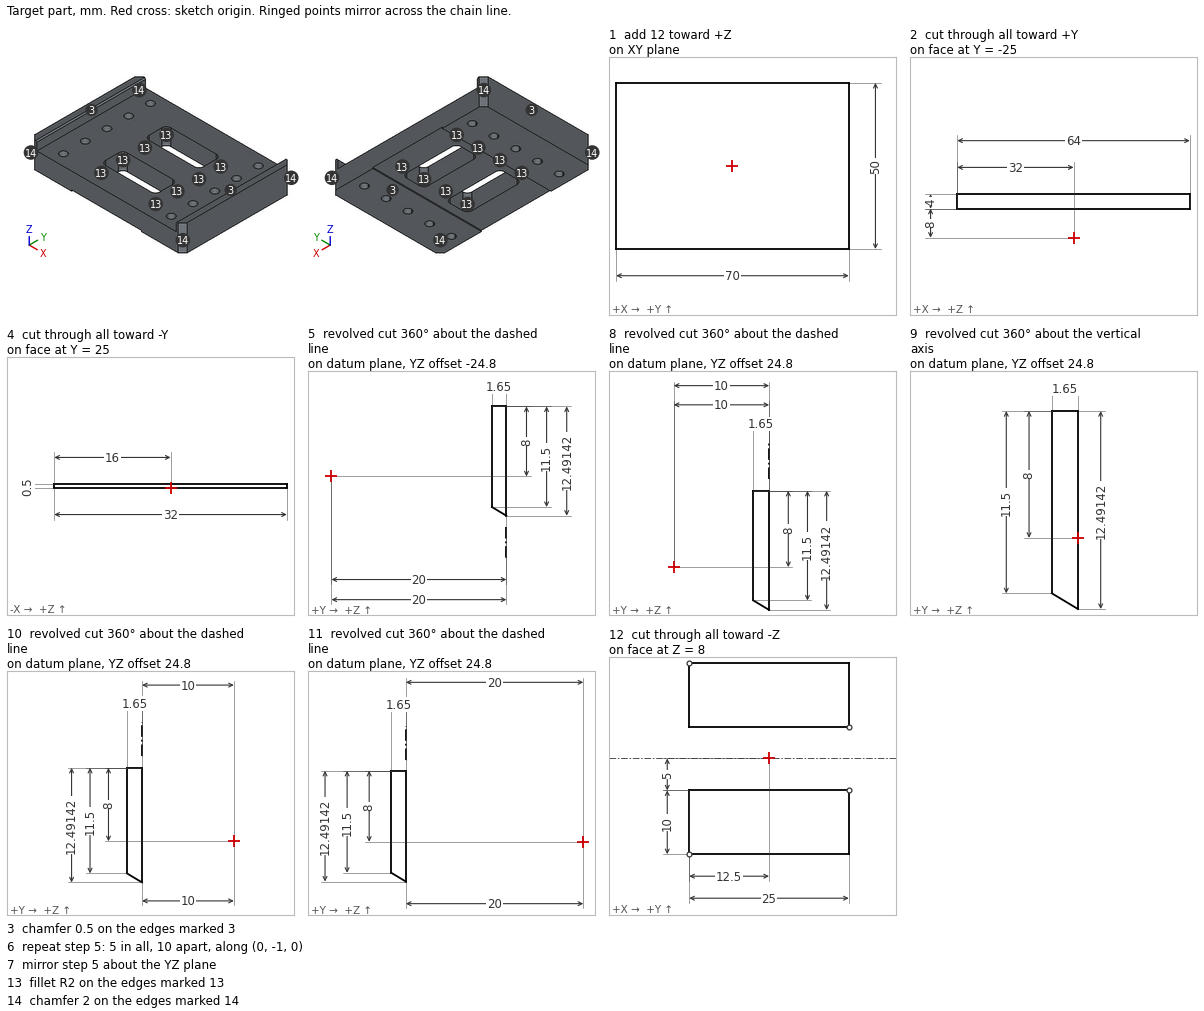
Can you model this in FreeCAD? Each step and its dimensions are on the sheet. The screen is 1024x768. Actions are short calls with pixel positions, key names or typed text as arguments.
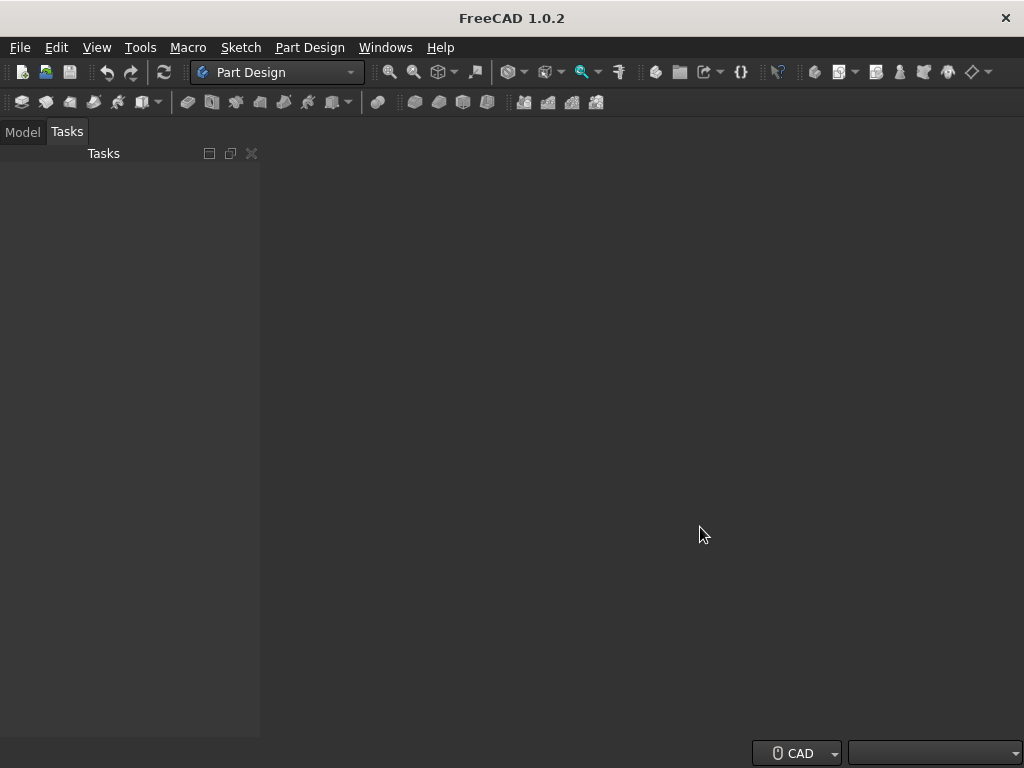
key(ctrl+n)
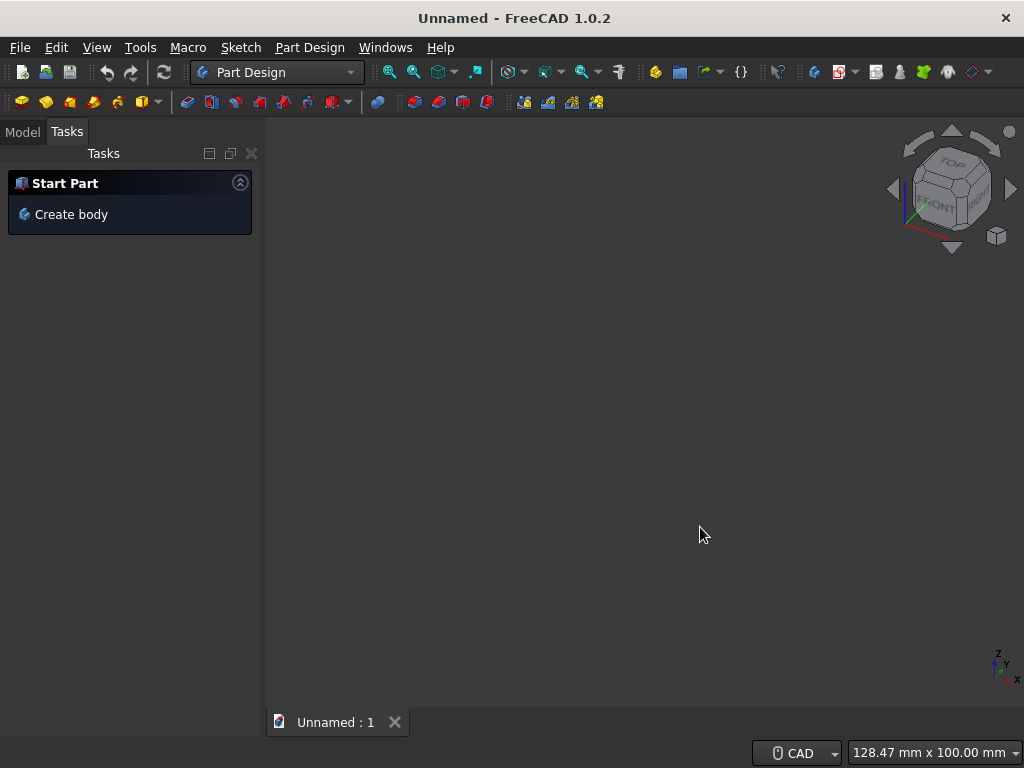
click(840, 72)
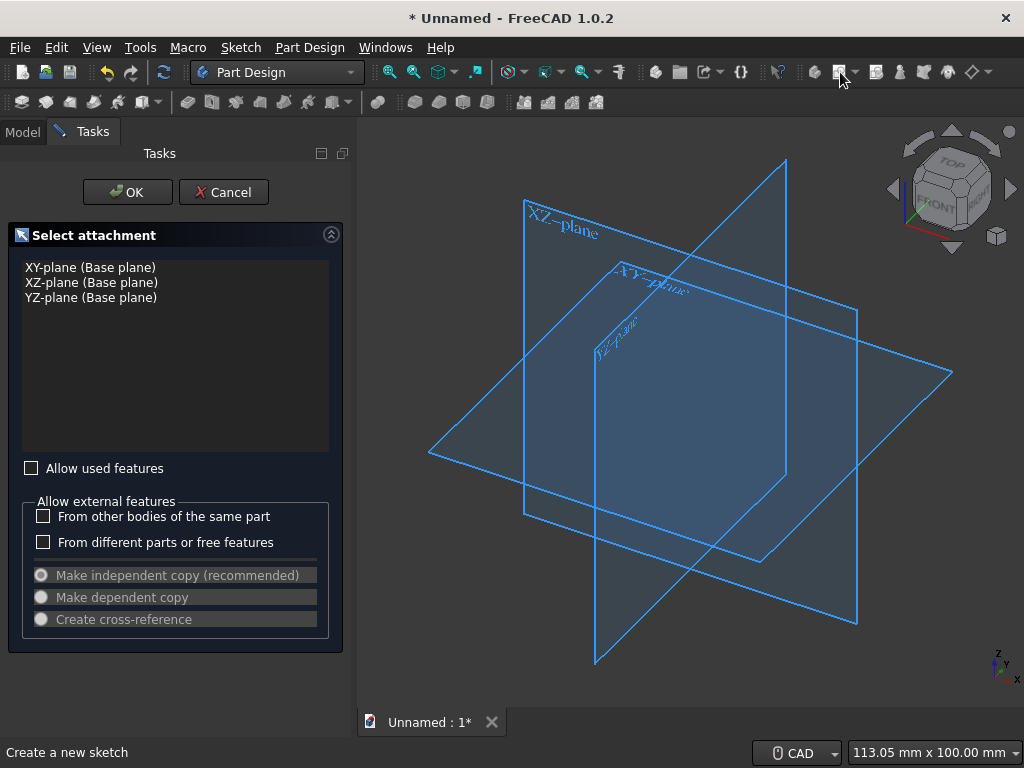
click(82, 268)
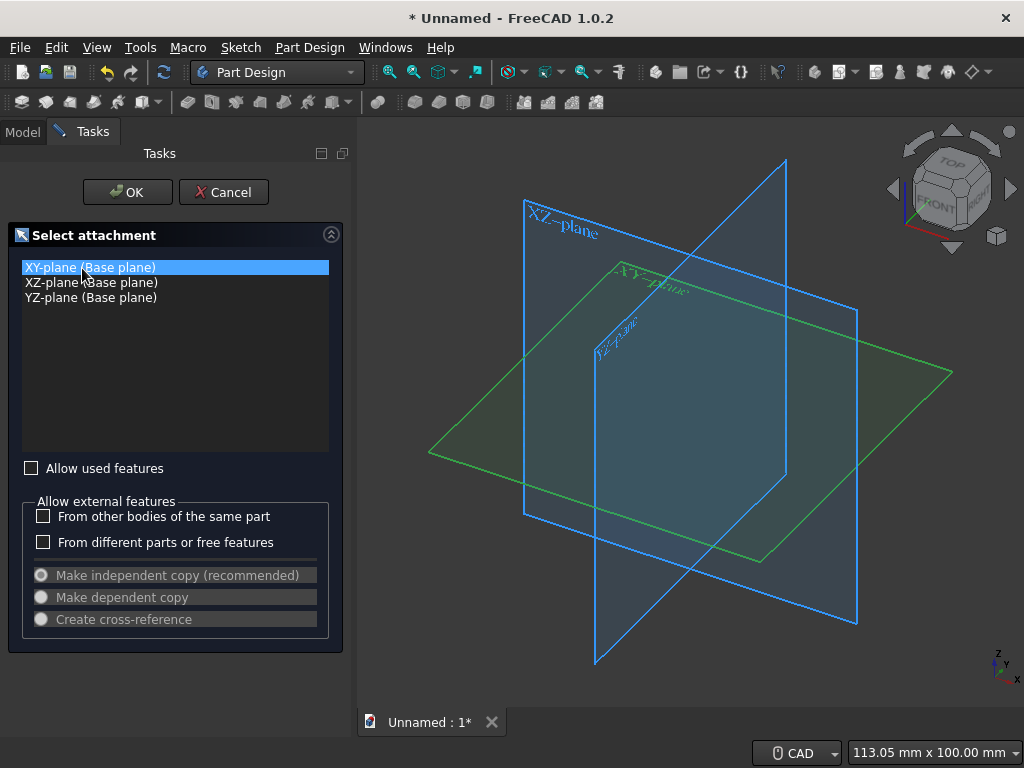
click(128, 192)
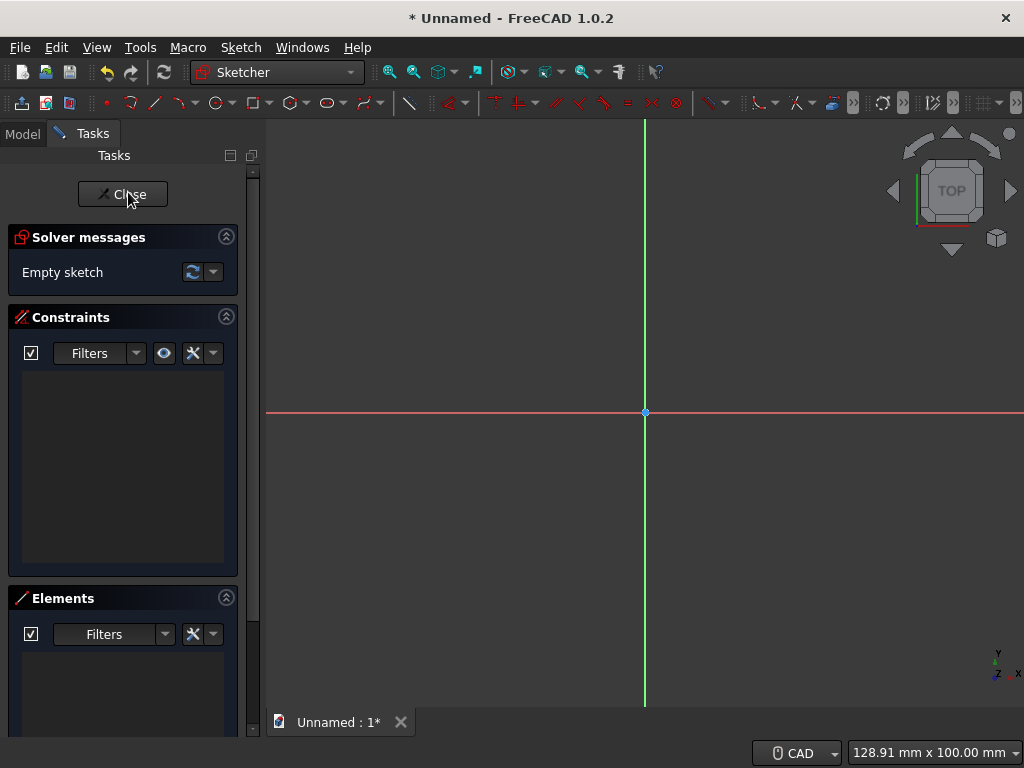
scroll(294, 413, down, 1)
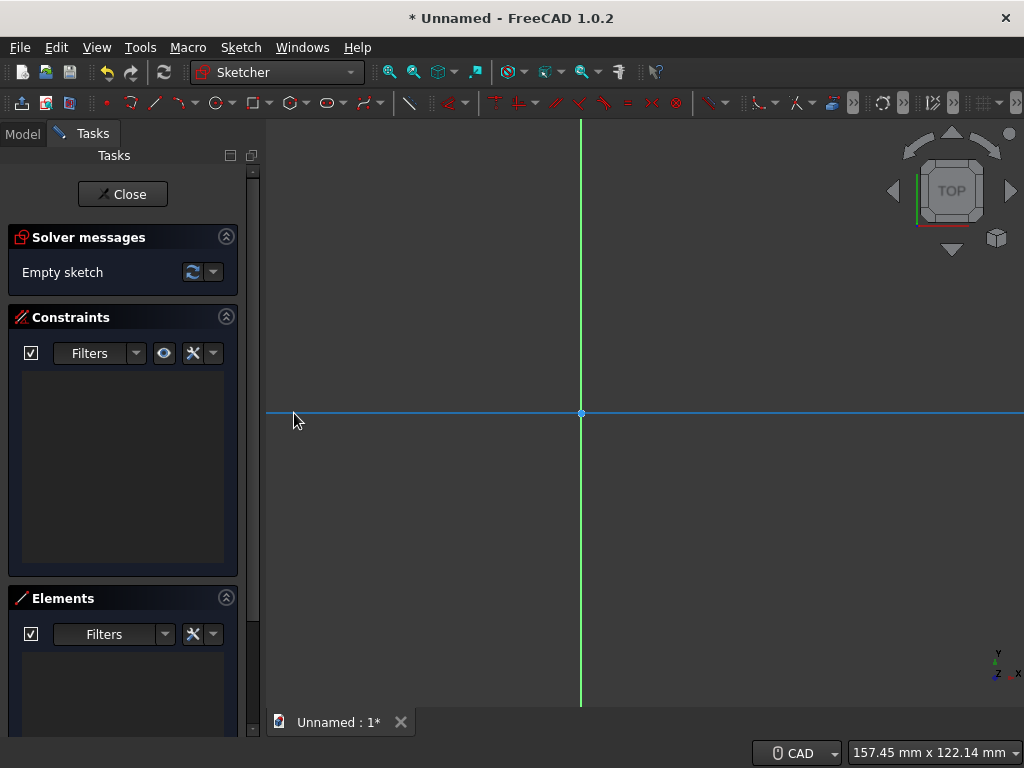
key(g)
key(v)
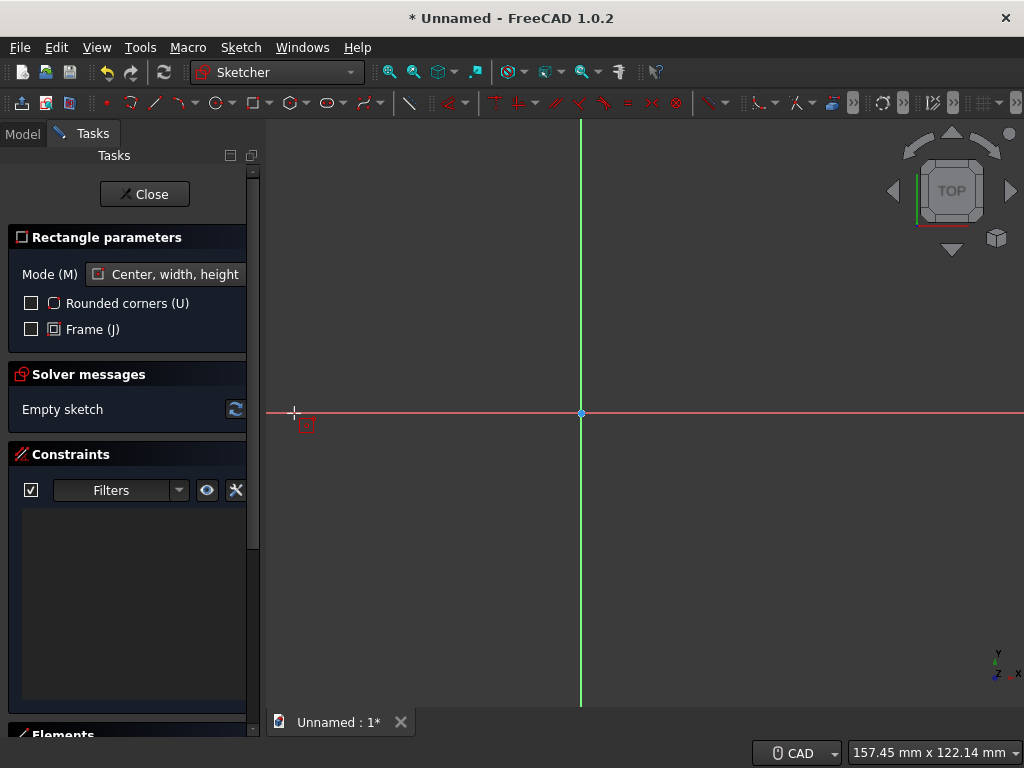
click(581, 413)
click(750, 293)
key(Escape)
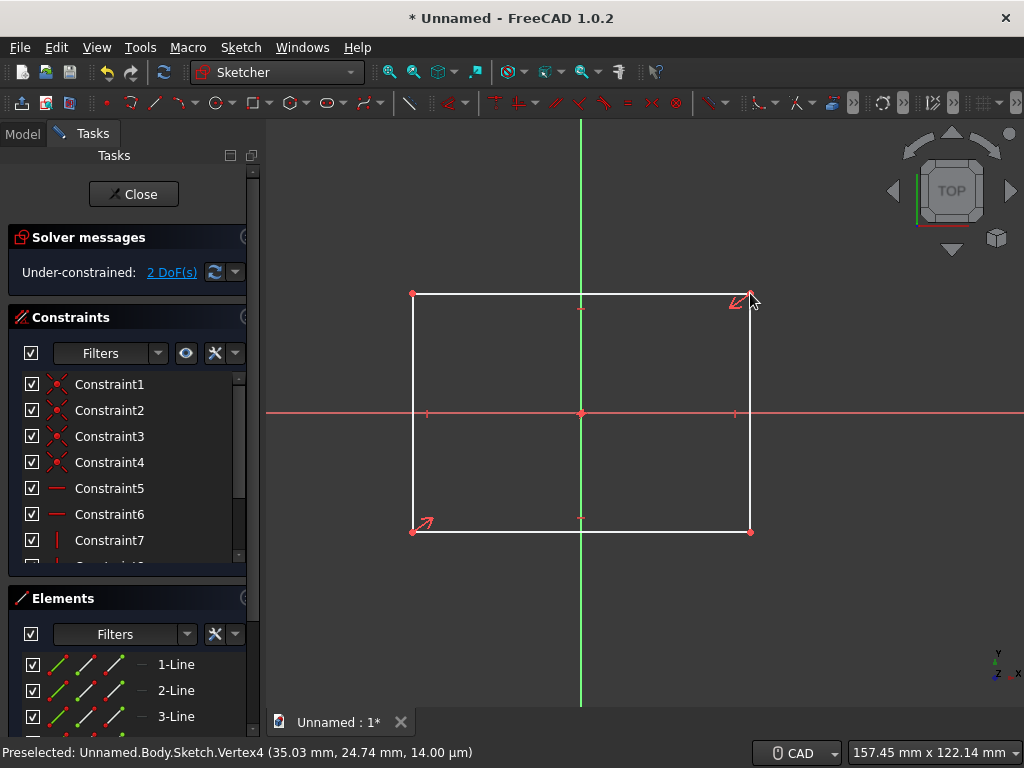
click(514, 532)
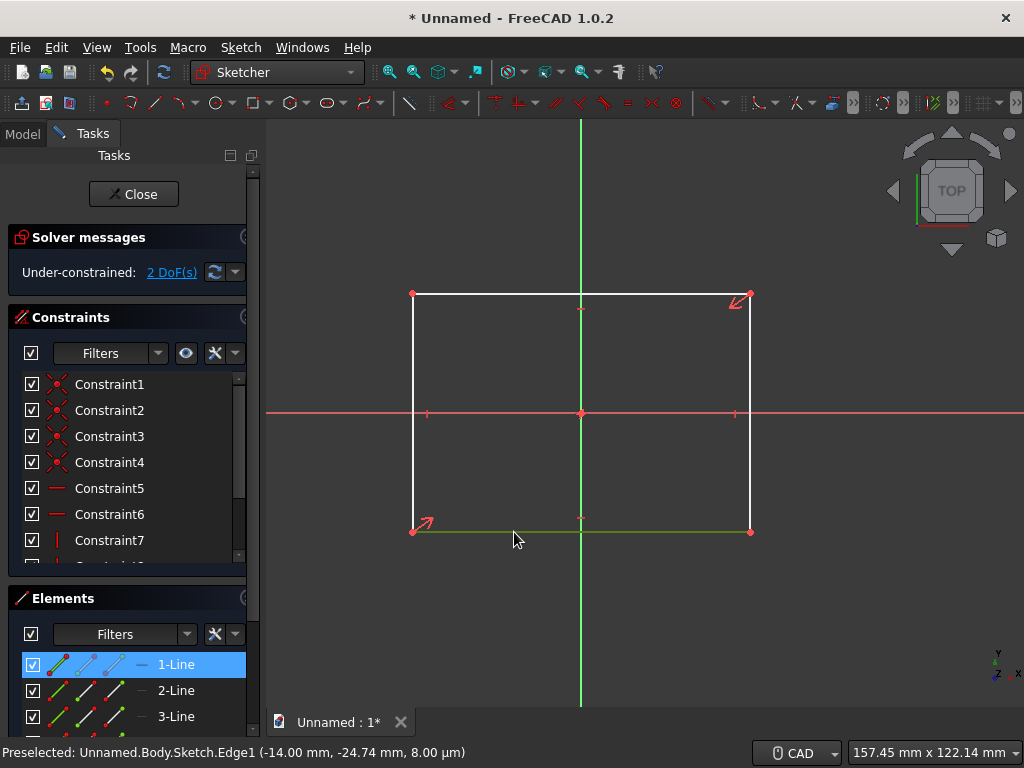
click(468, 104)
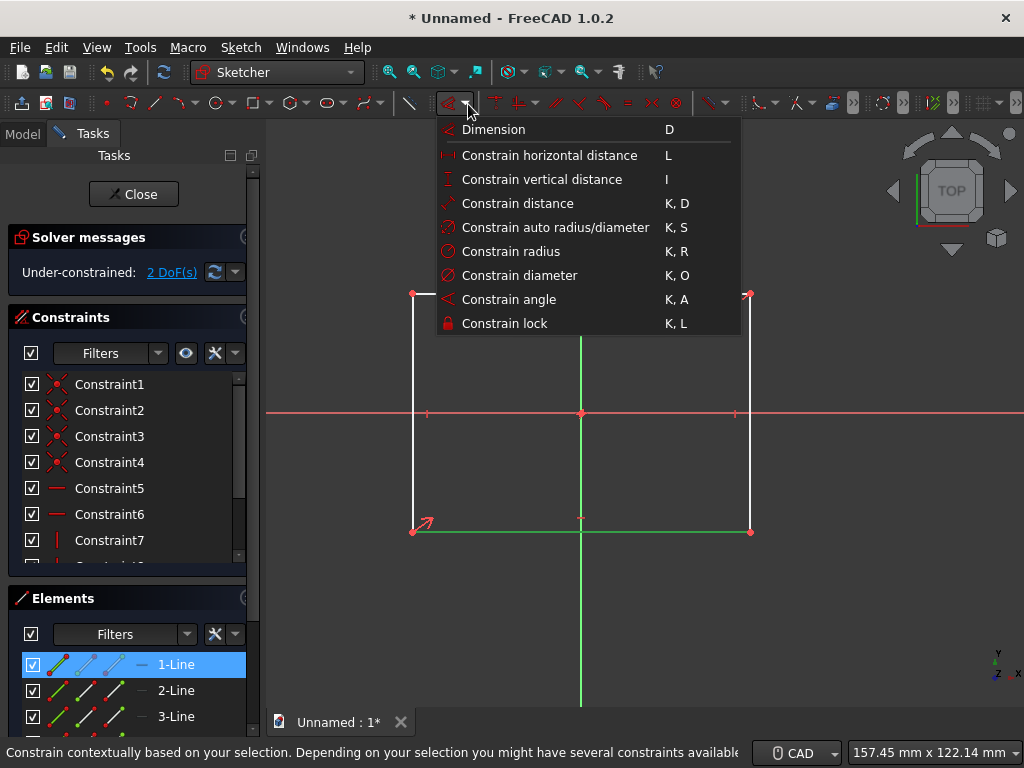
click(589, 155)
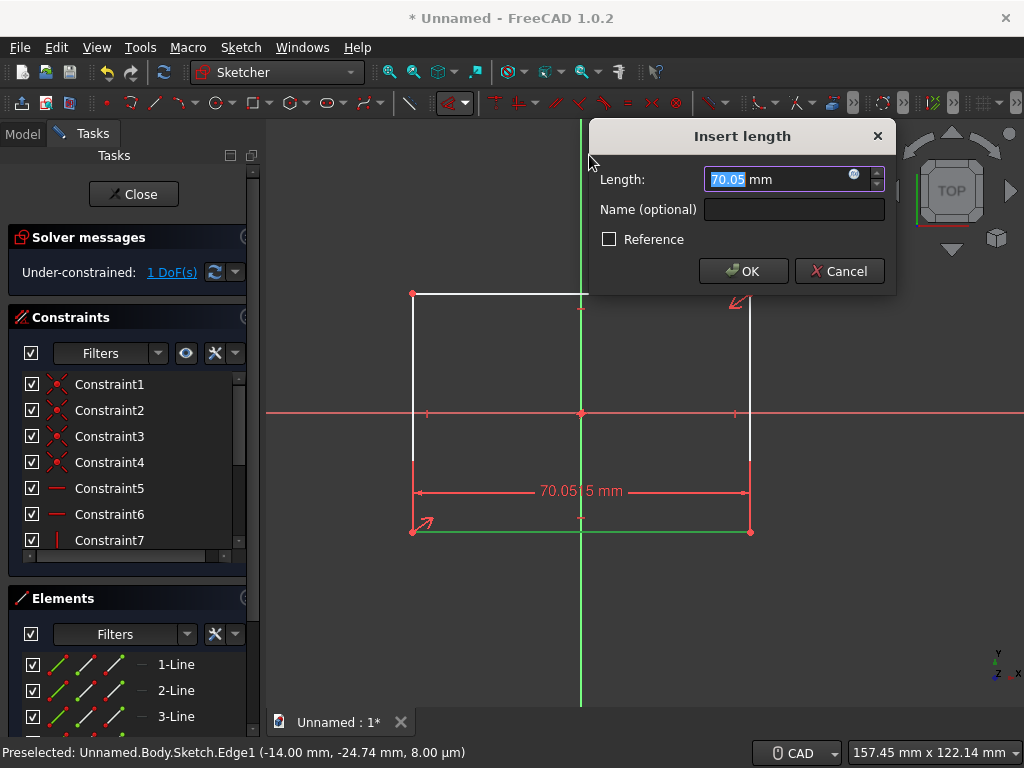
text(70)
key(Return)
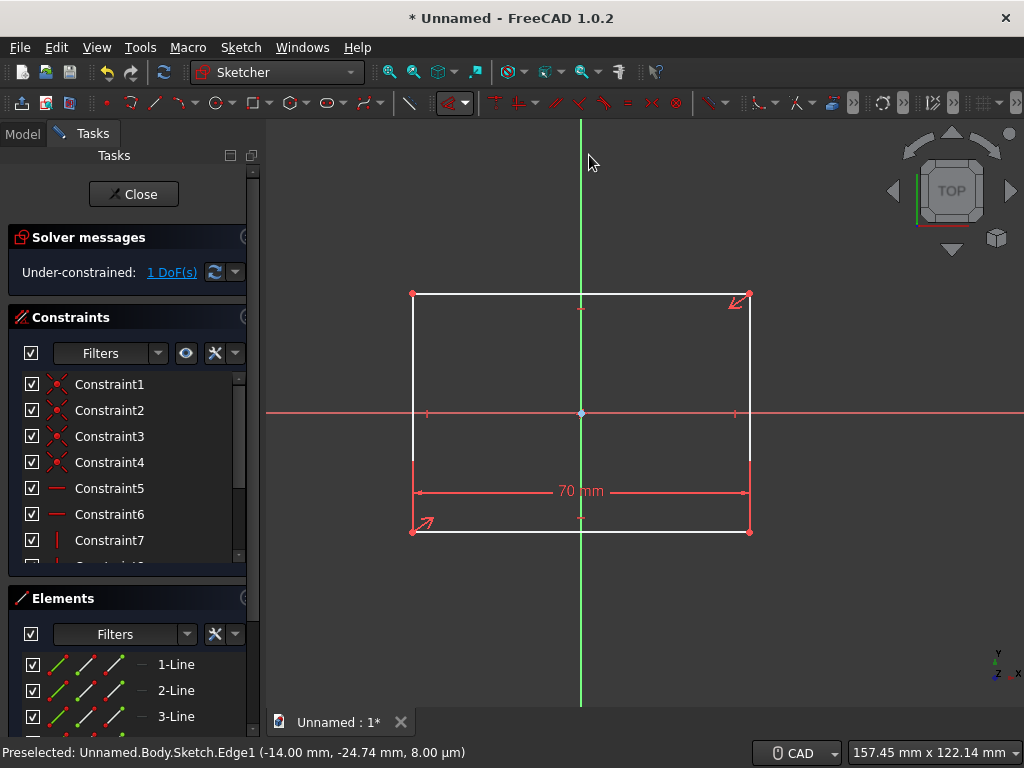
click(750, 461)